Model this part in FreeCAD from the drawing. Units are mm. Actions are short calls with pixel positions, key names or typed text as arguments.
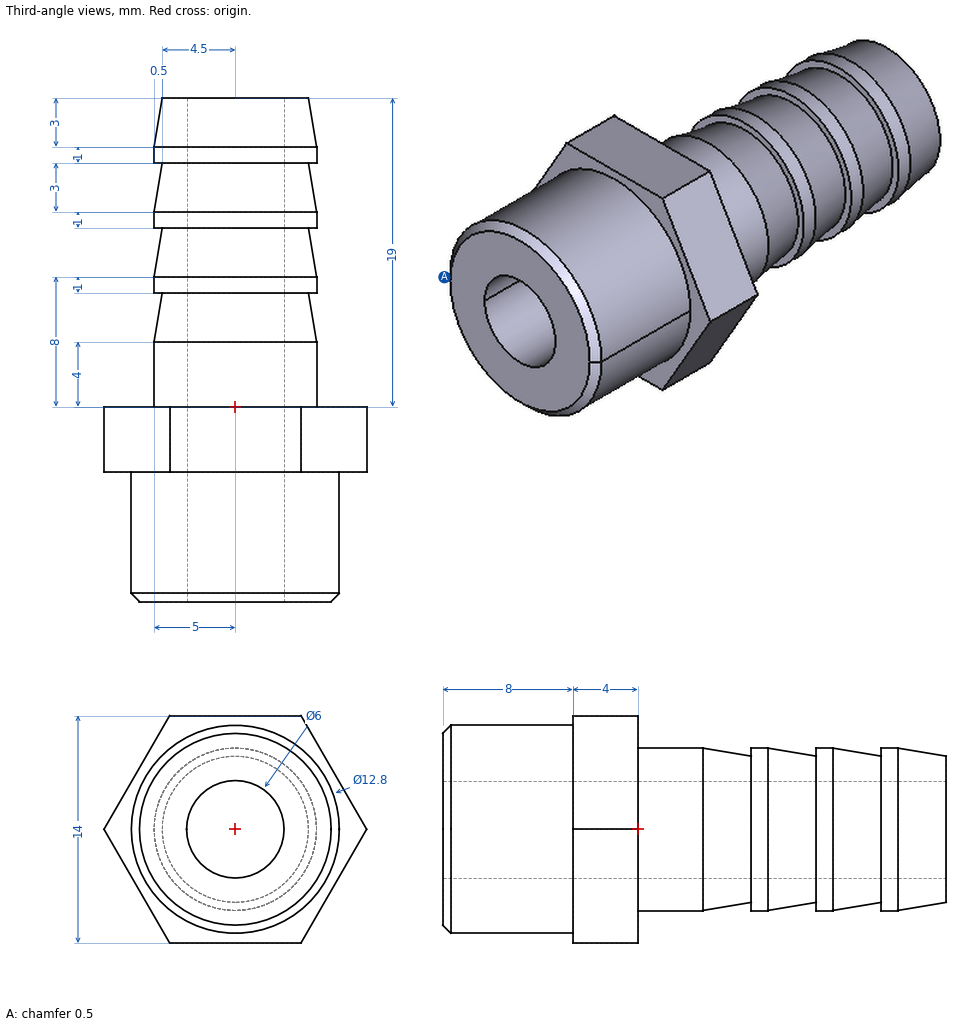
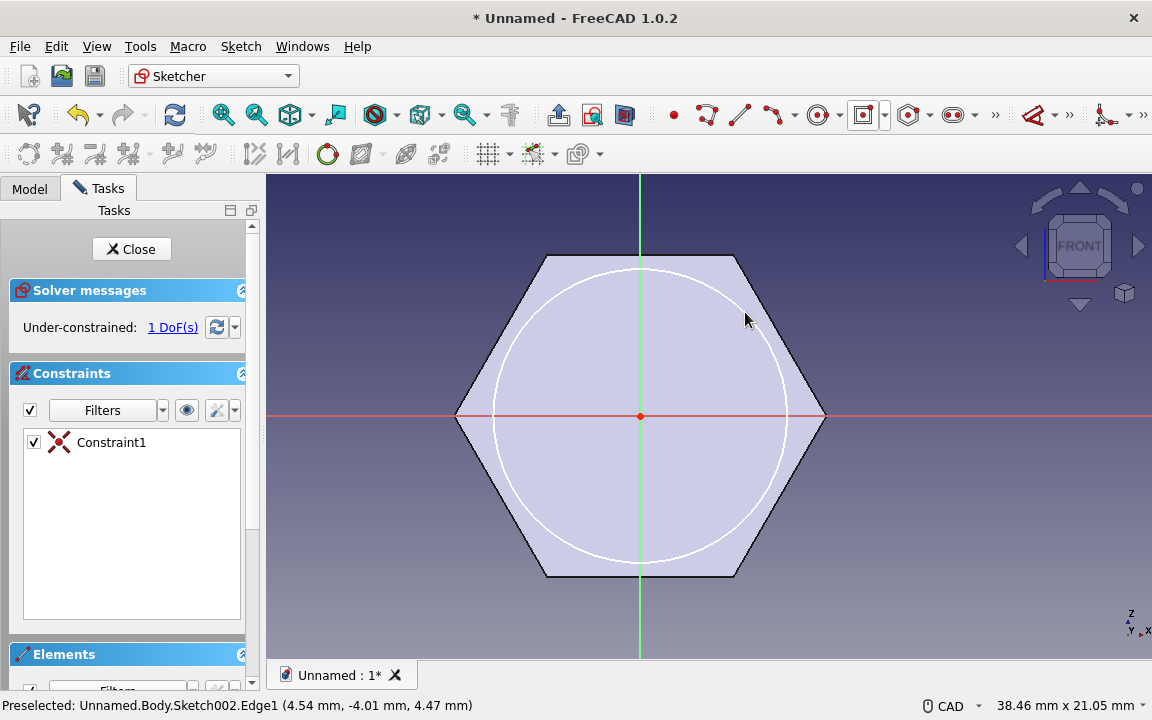
click(1032, 116)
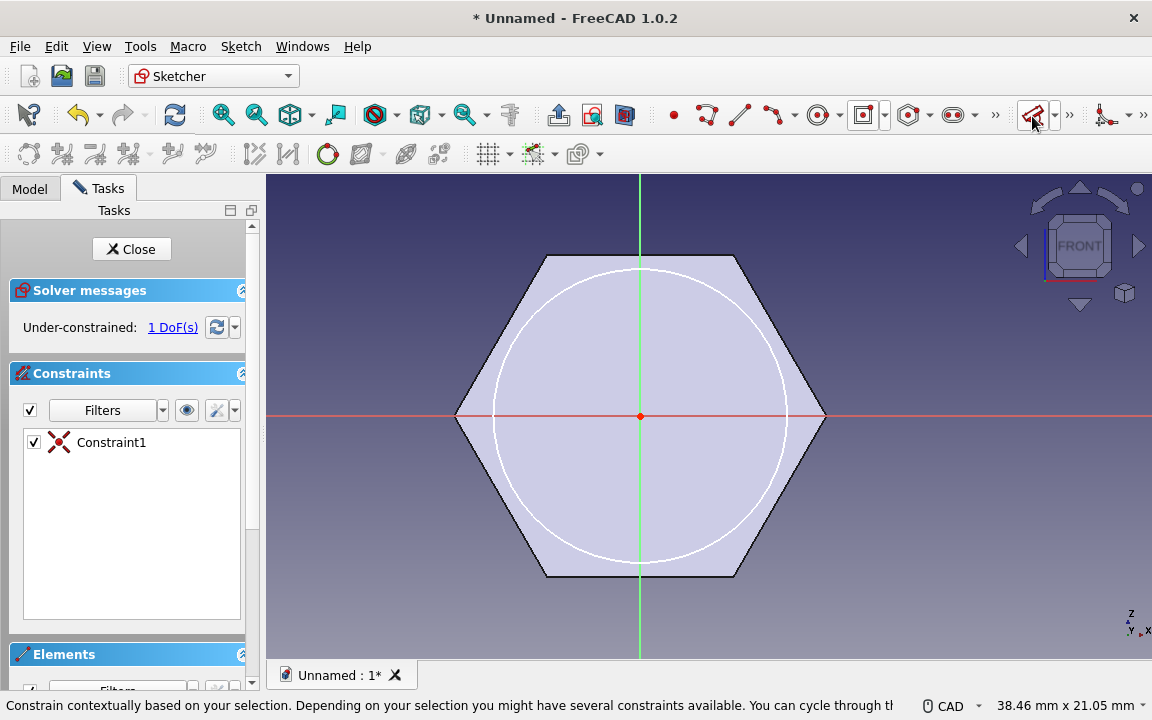
click(744, 312)
click(767, 289)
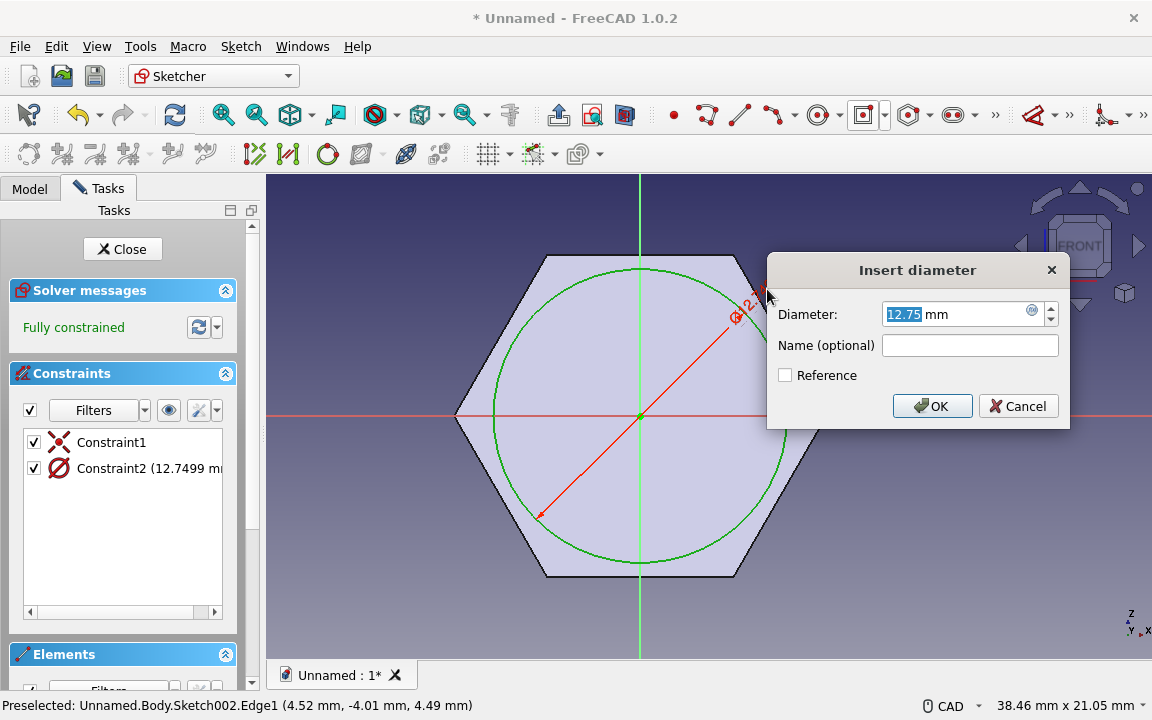
text(12.8)
key(Return)
key(Escape)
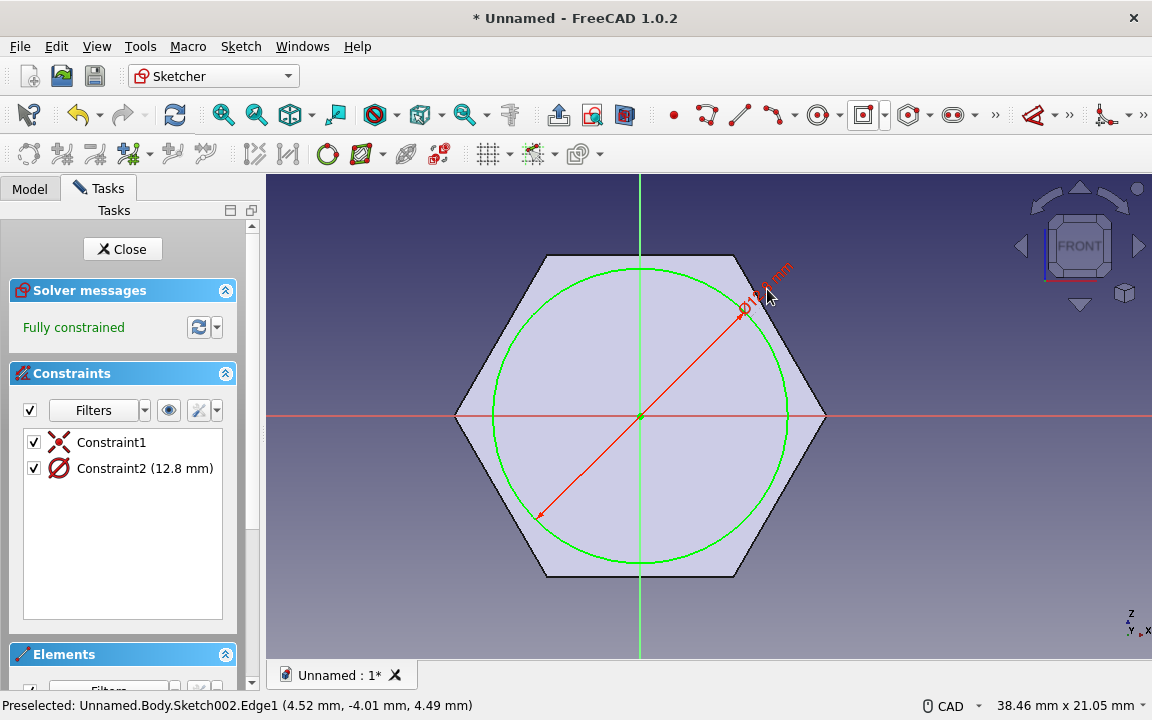
click(123, 249)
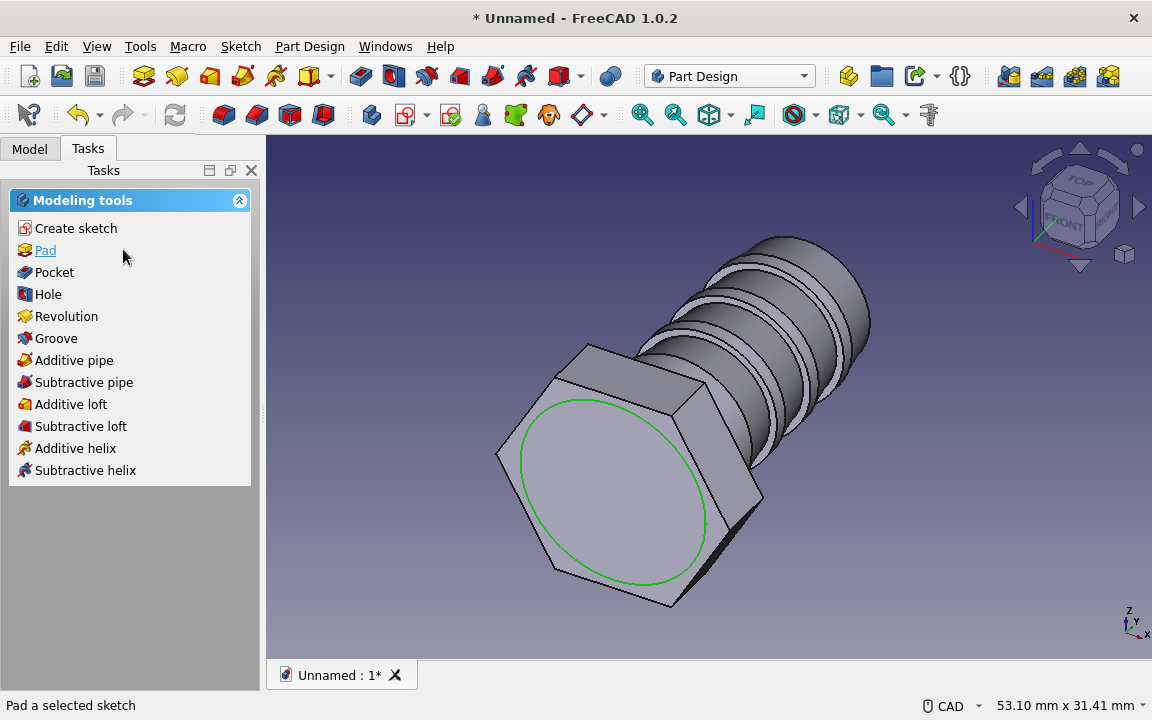
click(144, 76)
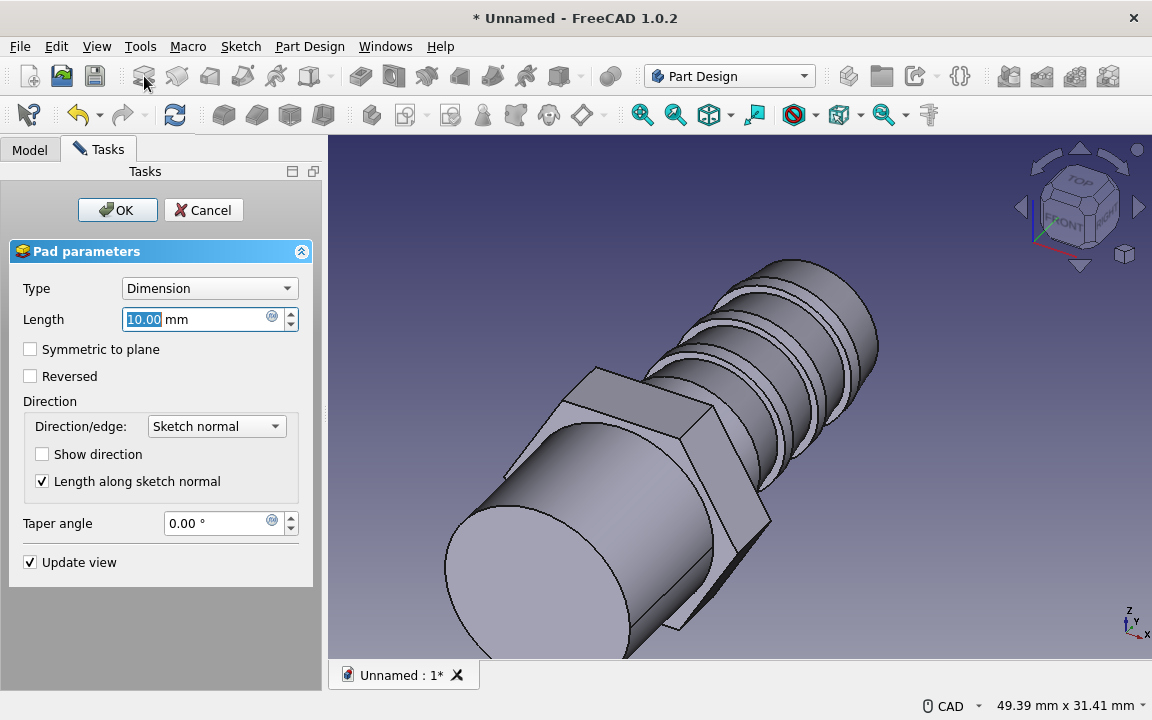
text(8)
key(Tab)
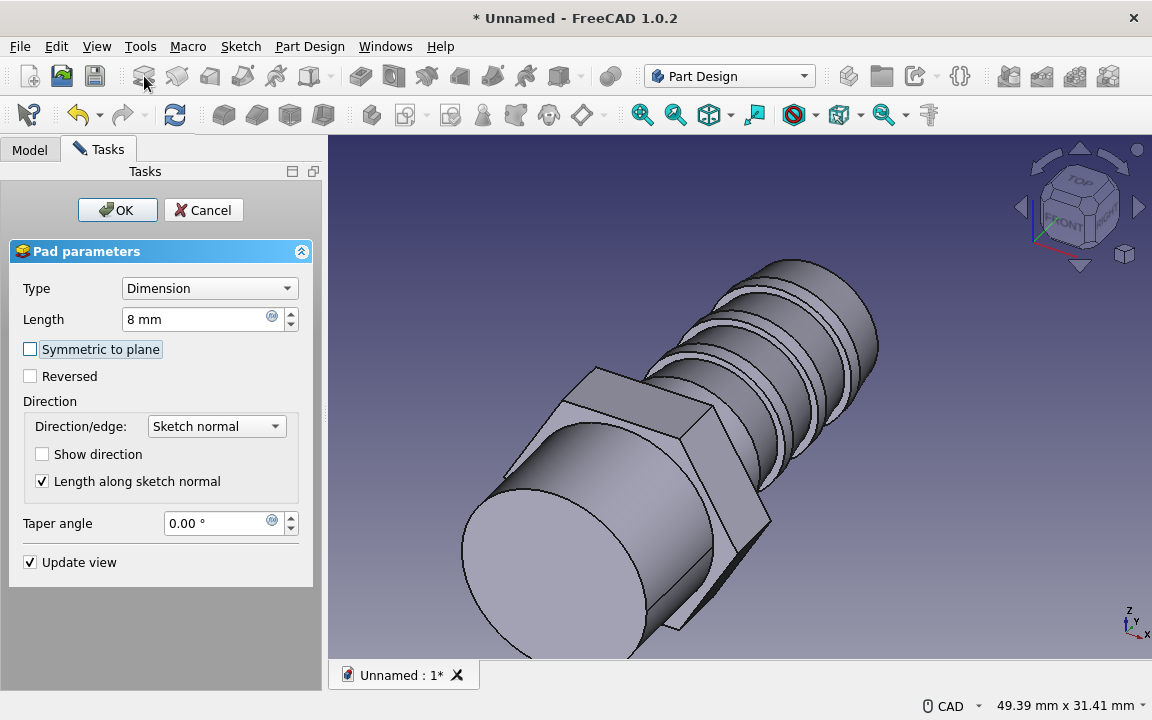
click(118, 210)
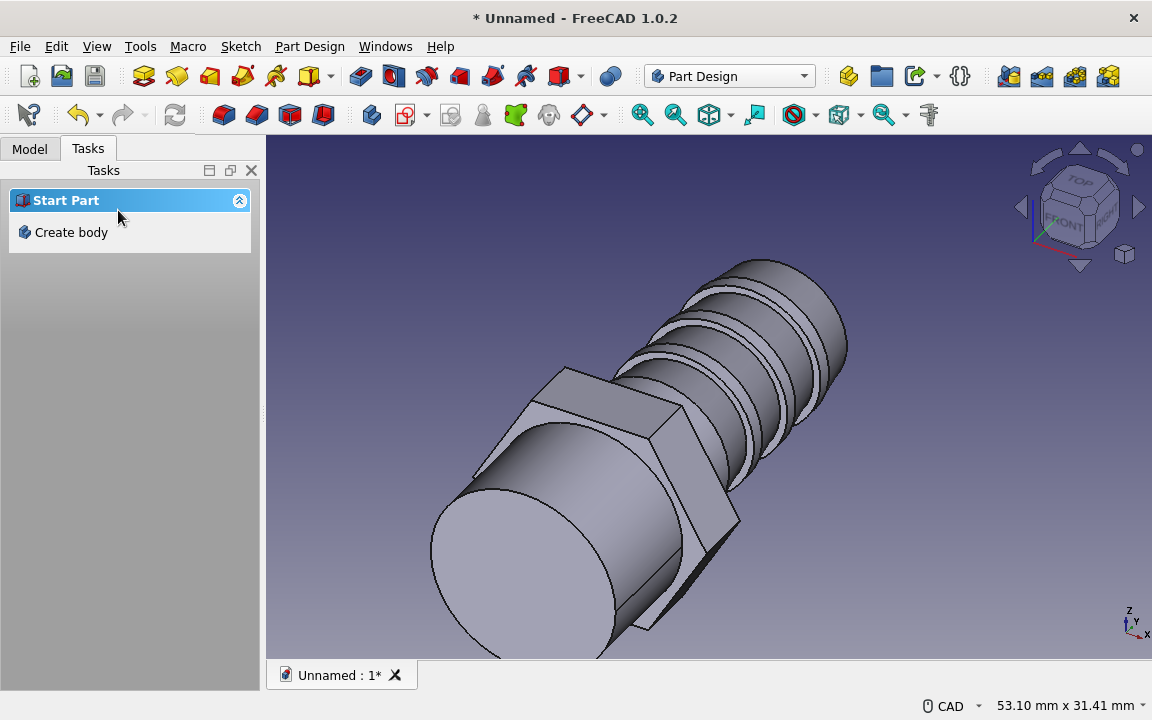
click(643, 116)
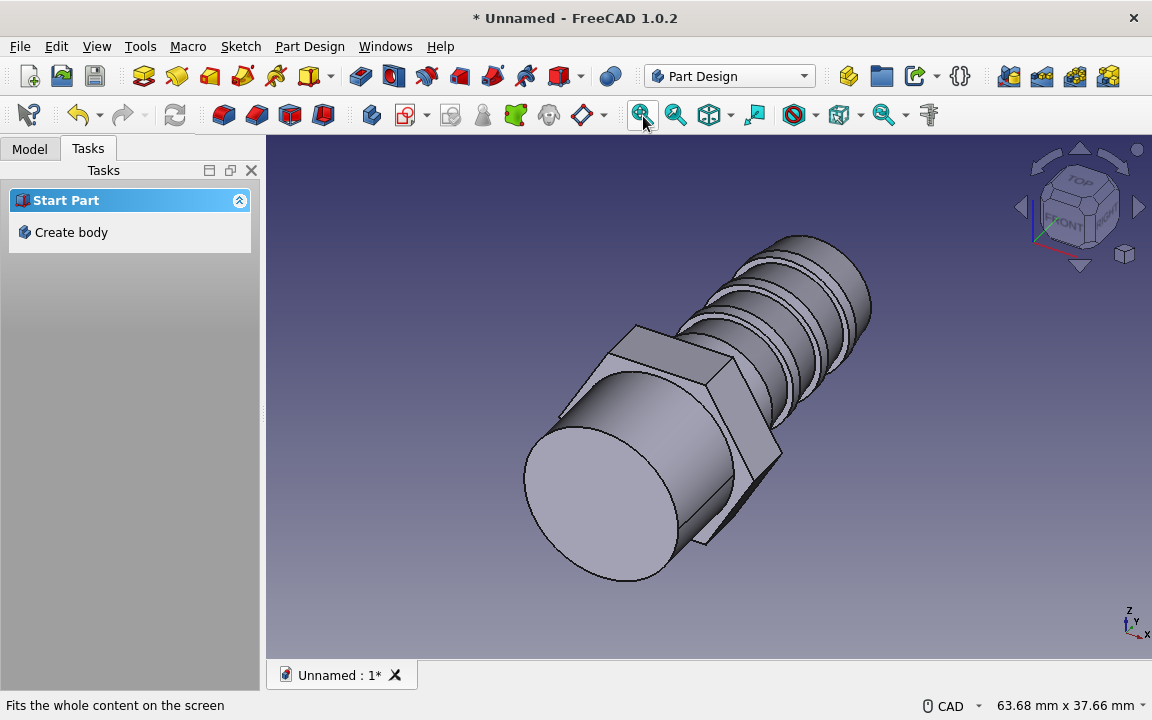
key(4)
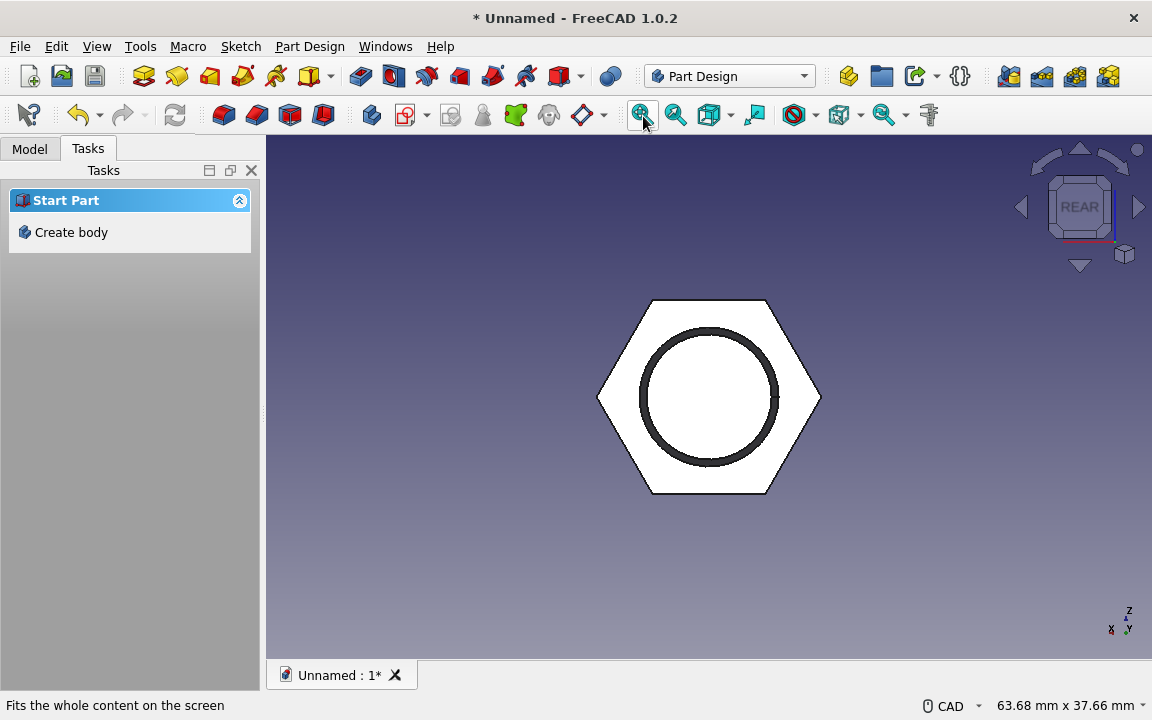
click(643, 116)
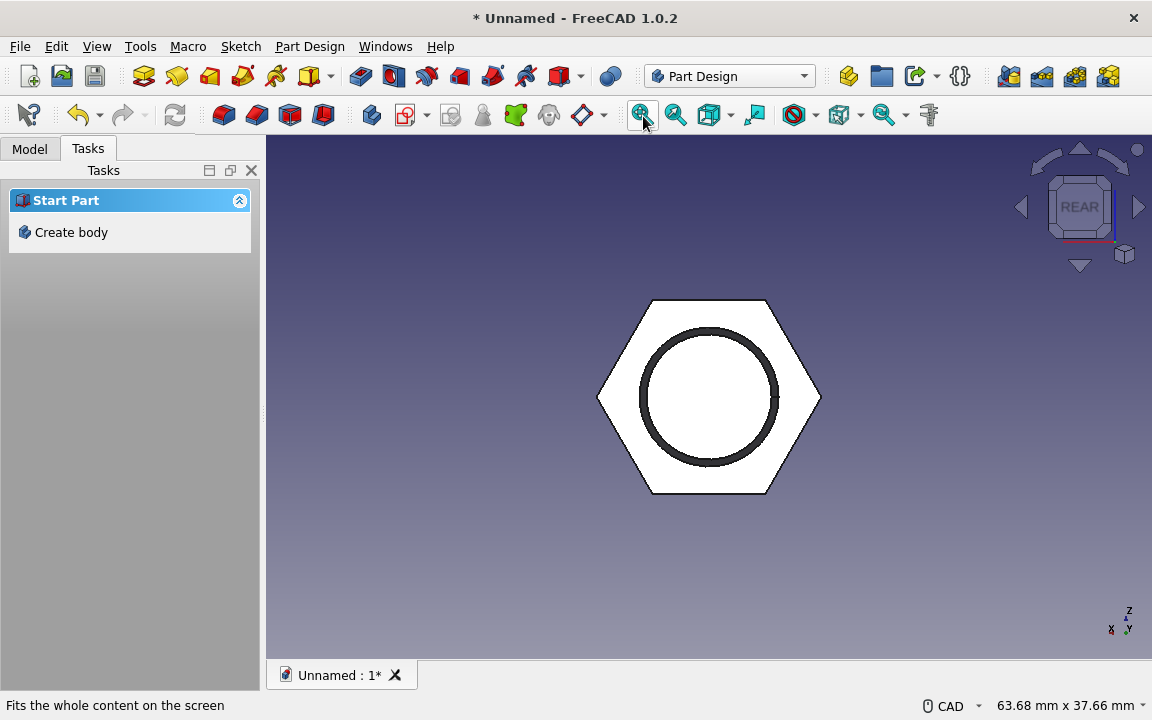
click(709, 396)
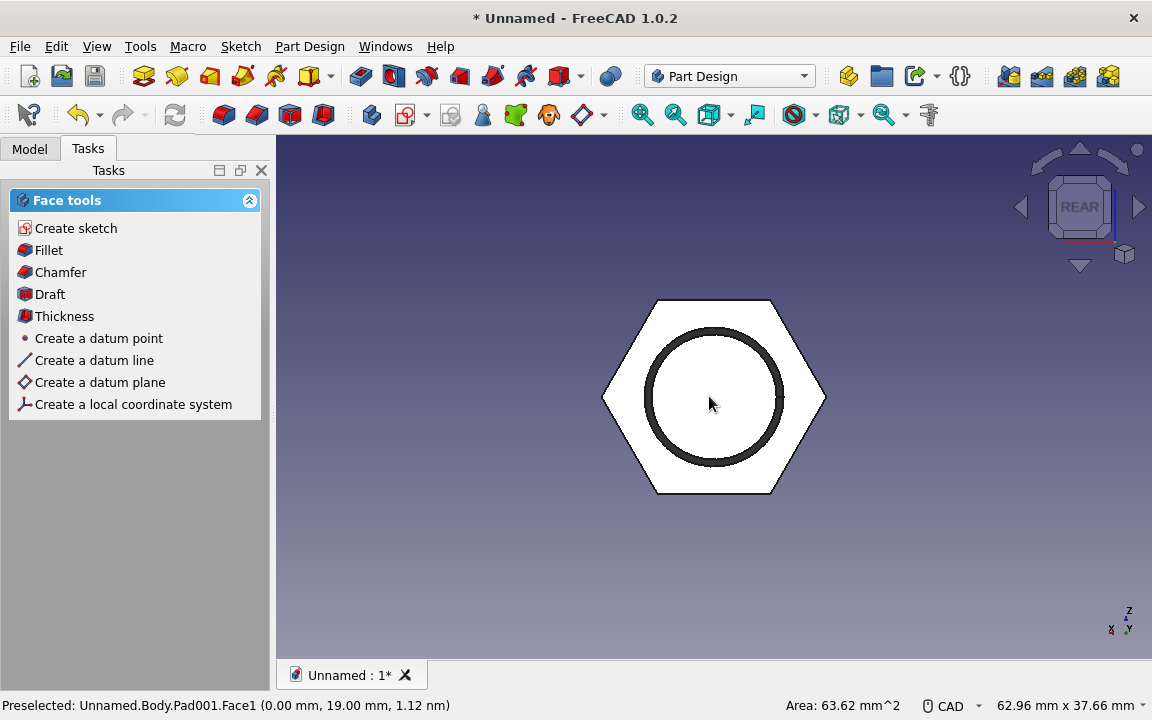
click(404, 116)